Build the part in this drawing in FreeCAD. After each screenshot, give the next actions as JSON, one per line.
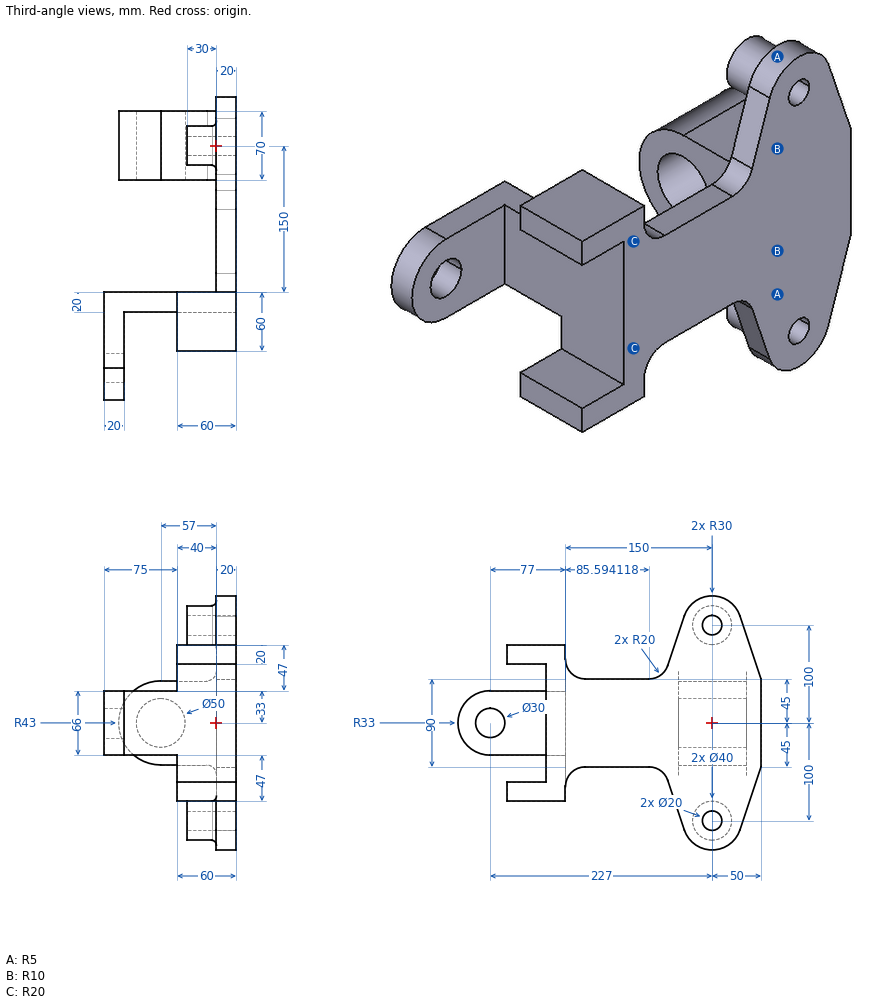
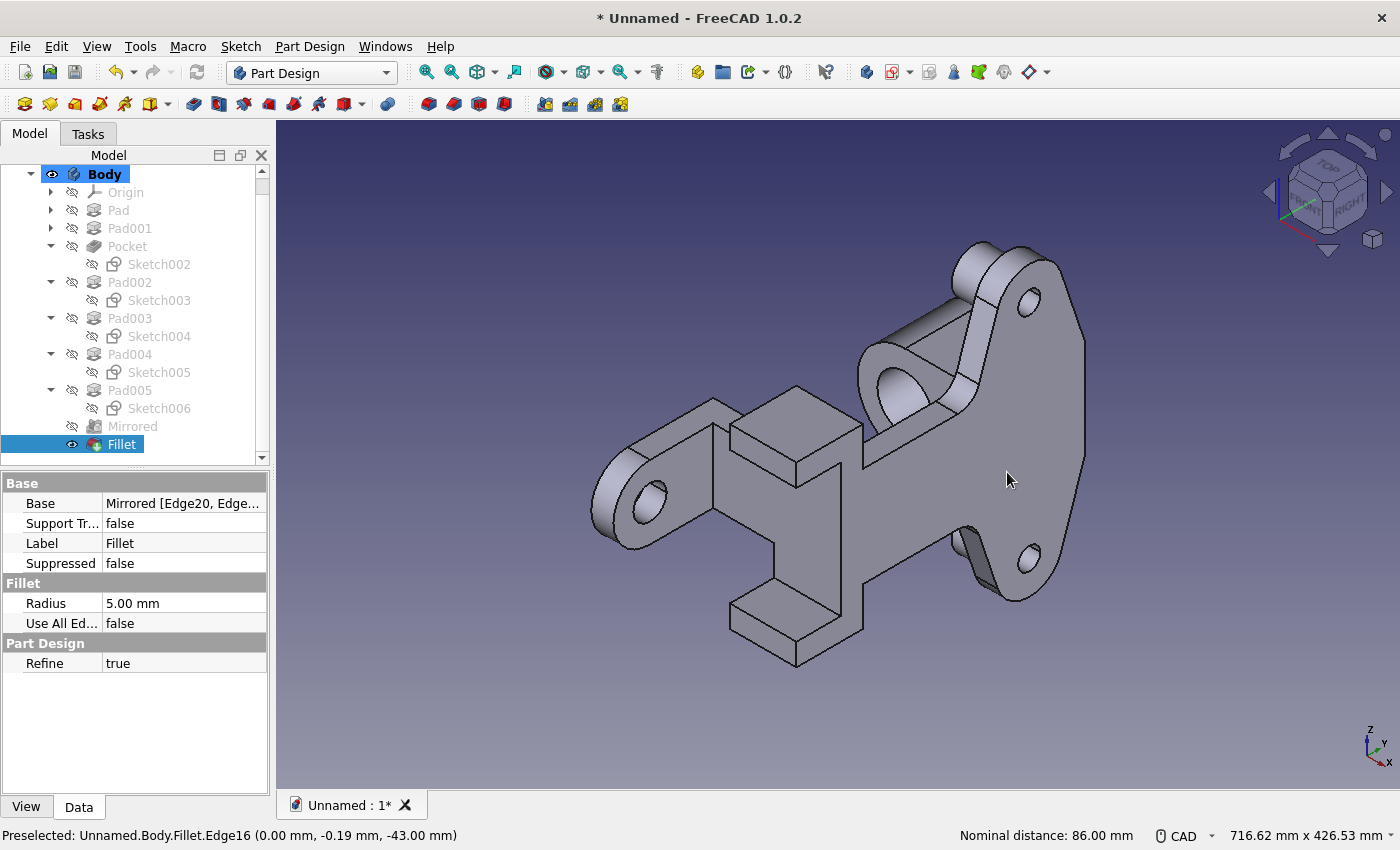
{"action": "left_click", "coordinate": [429, 104]}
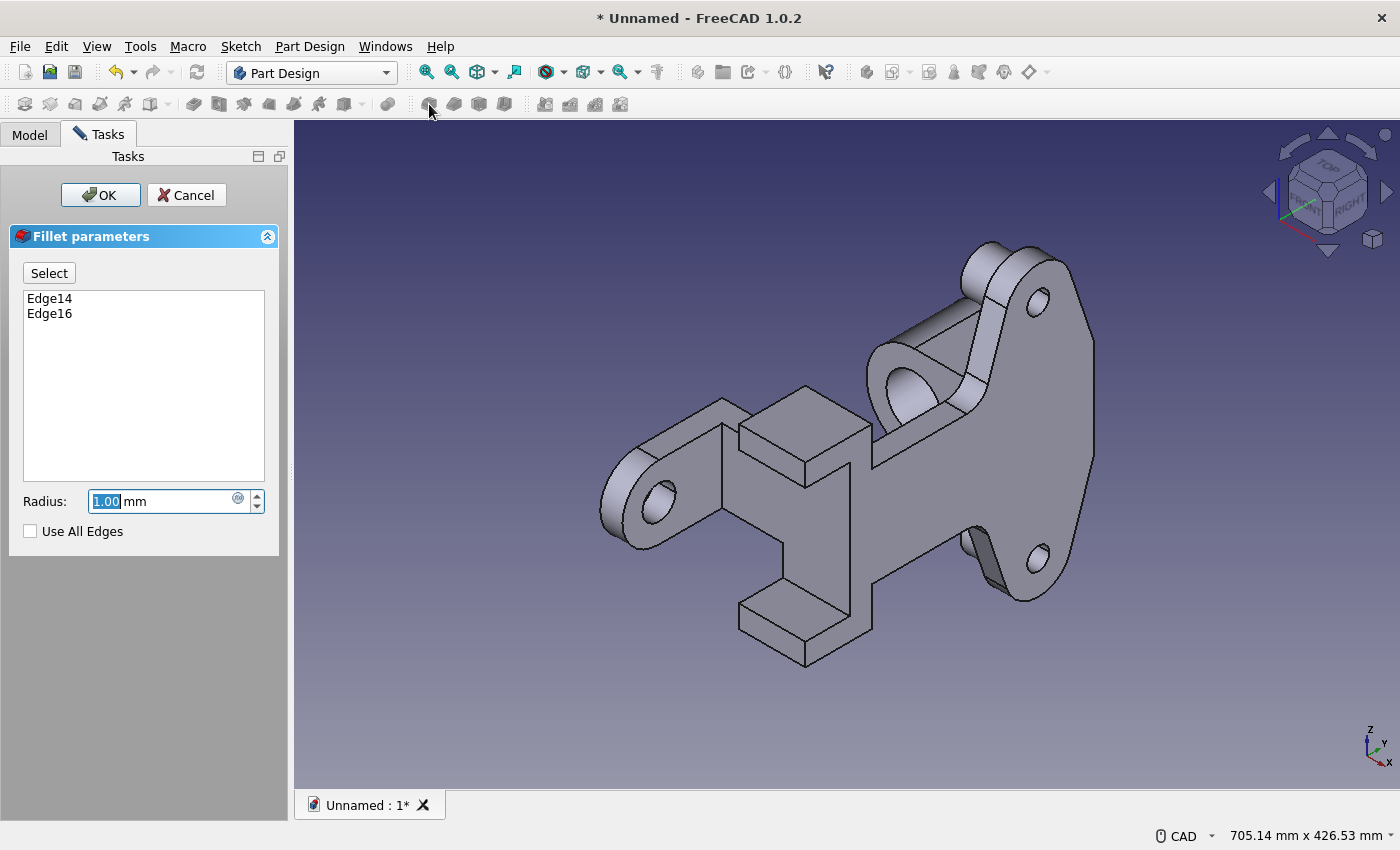
{"action": "type", "text": "10"}
{"action": "key", "text": "Tab"}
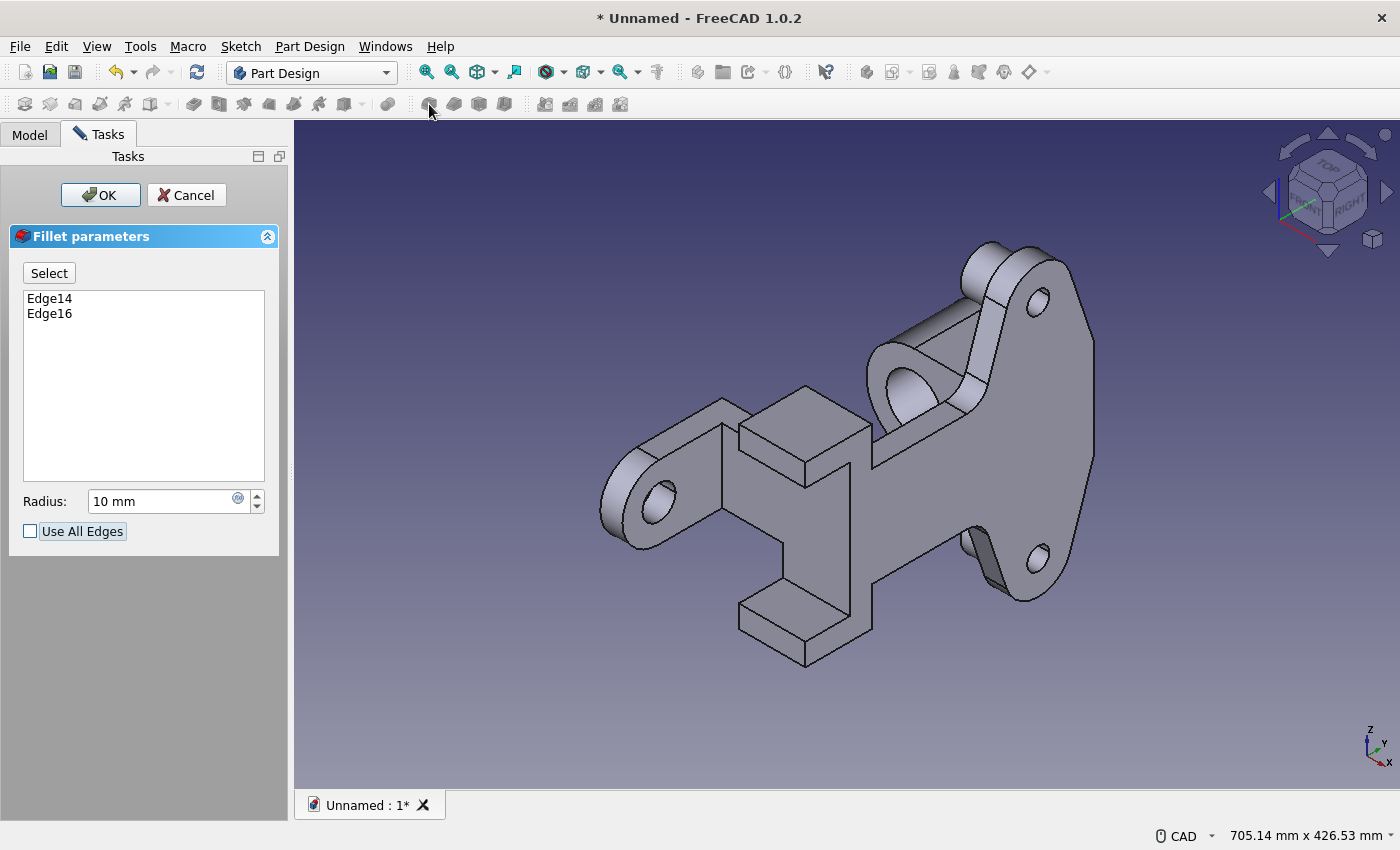
{"action": "left_click", "coordinate": [101, 195]}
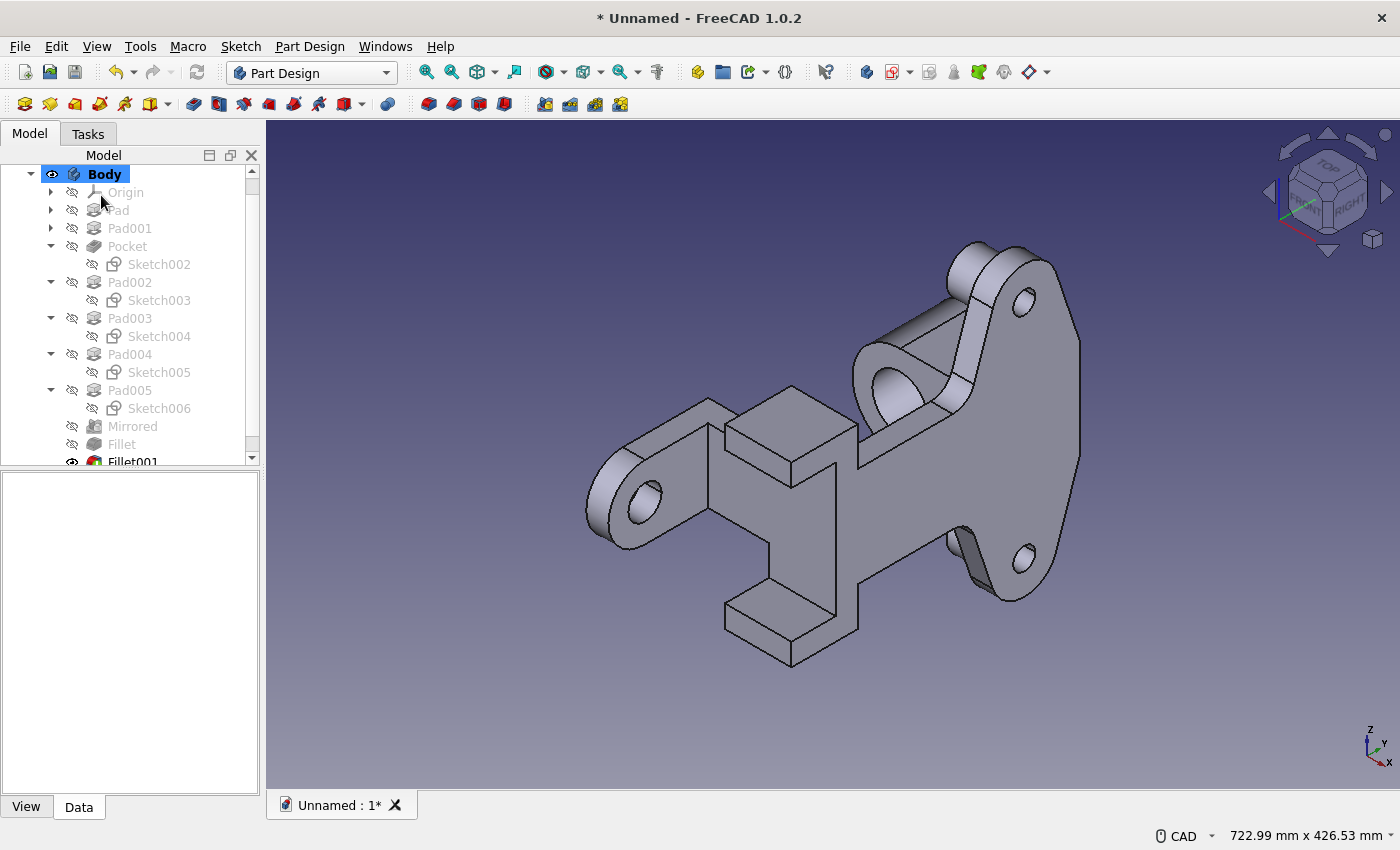
{"action": "key", "text": "2"}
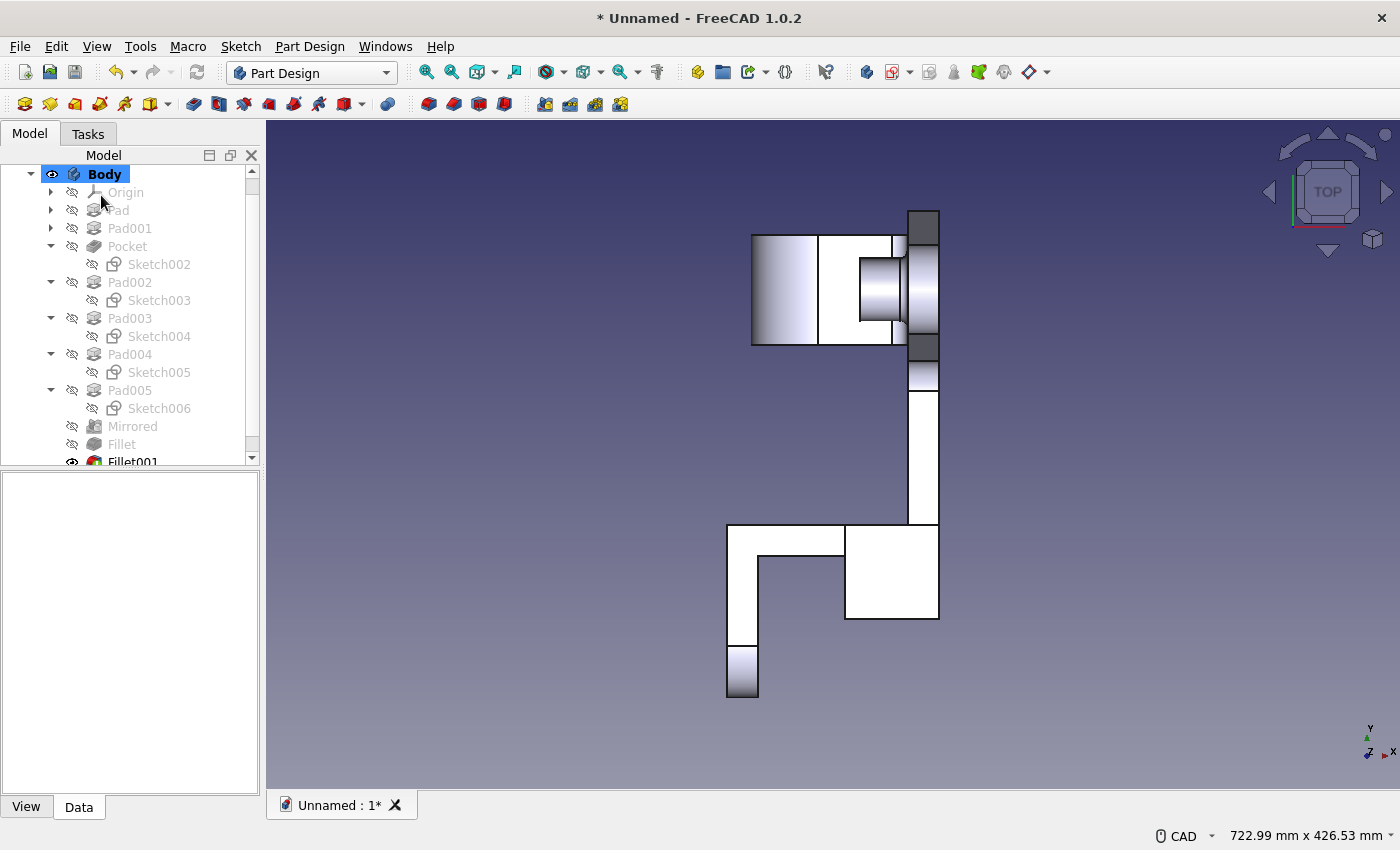
{"action": "key", "text": "0"}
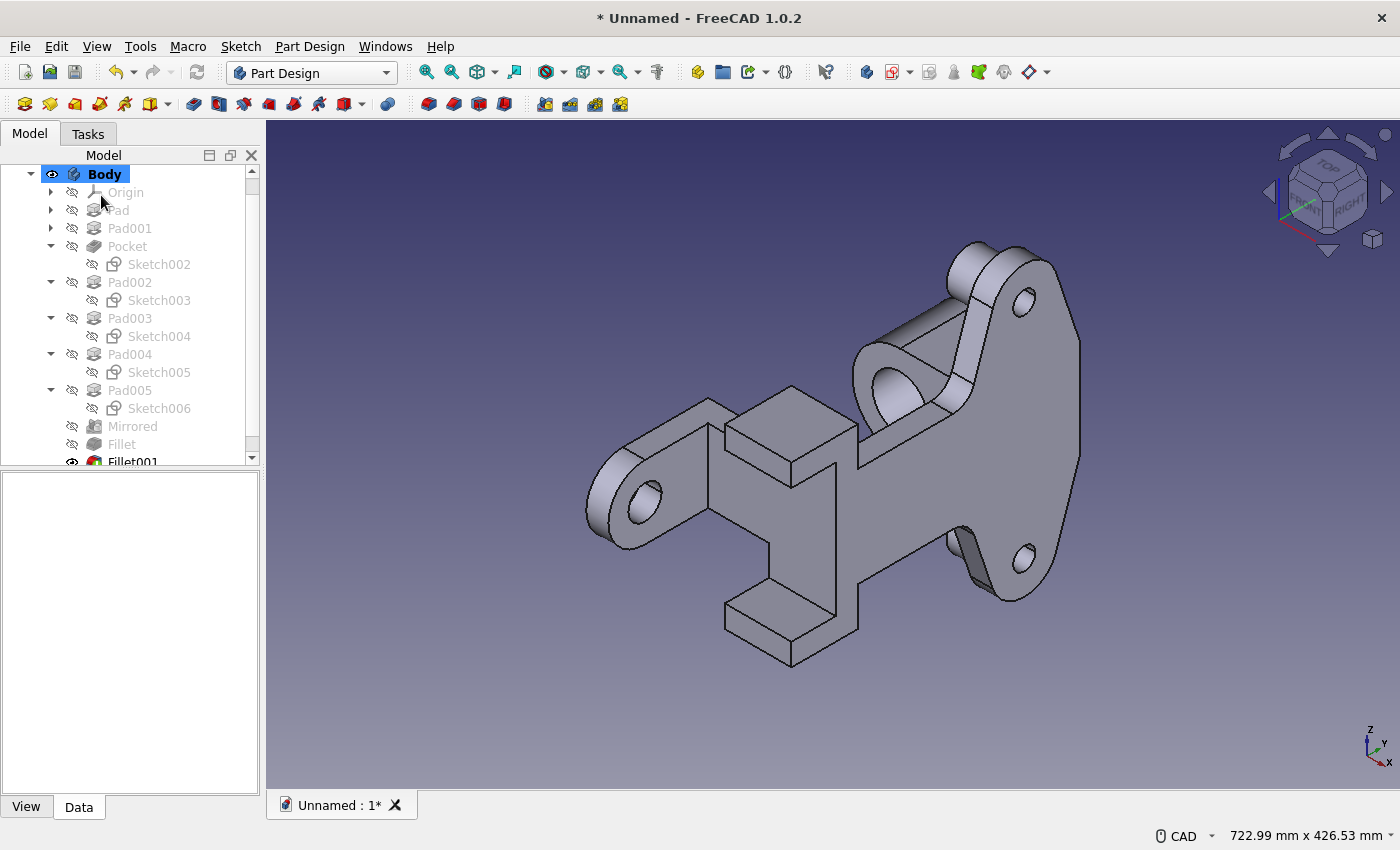
{"action": "key", "text": "1"}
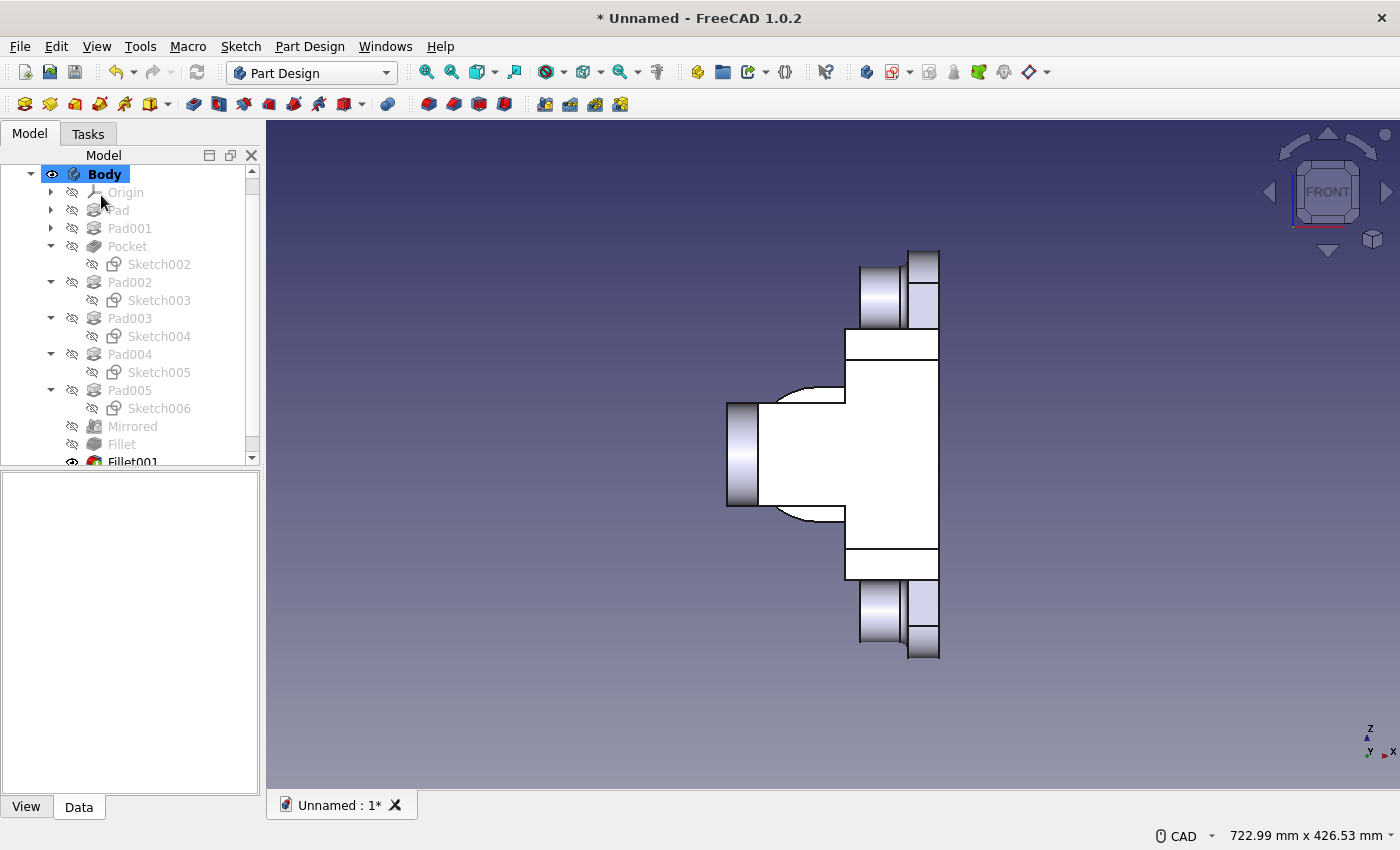
{"action": "key", "text": "3"}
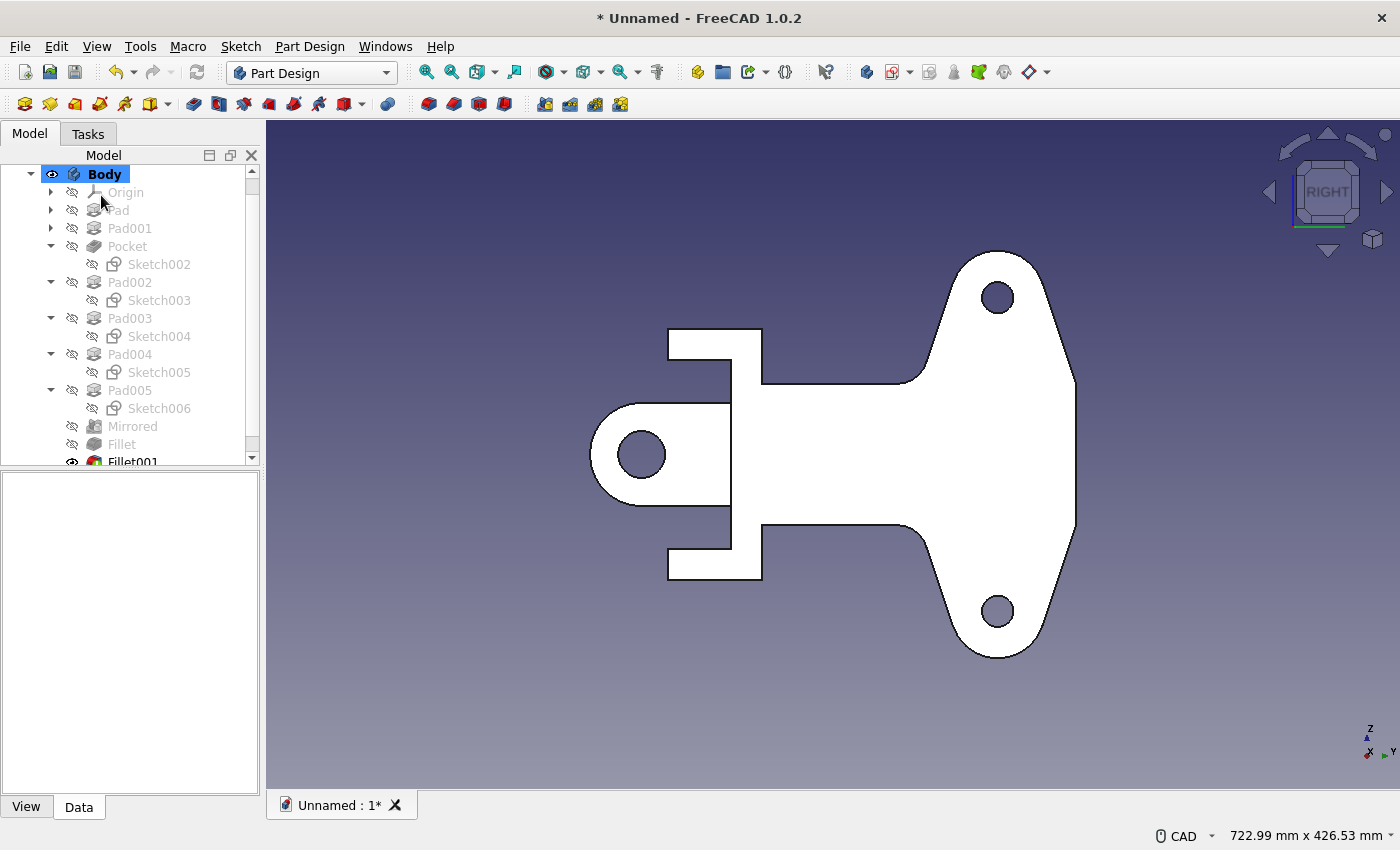
{"action": "key", "text": "5"}